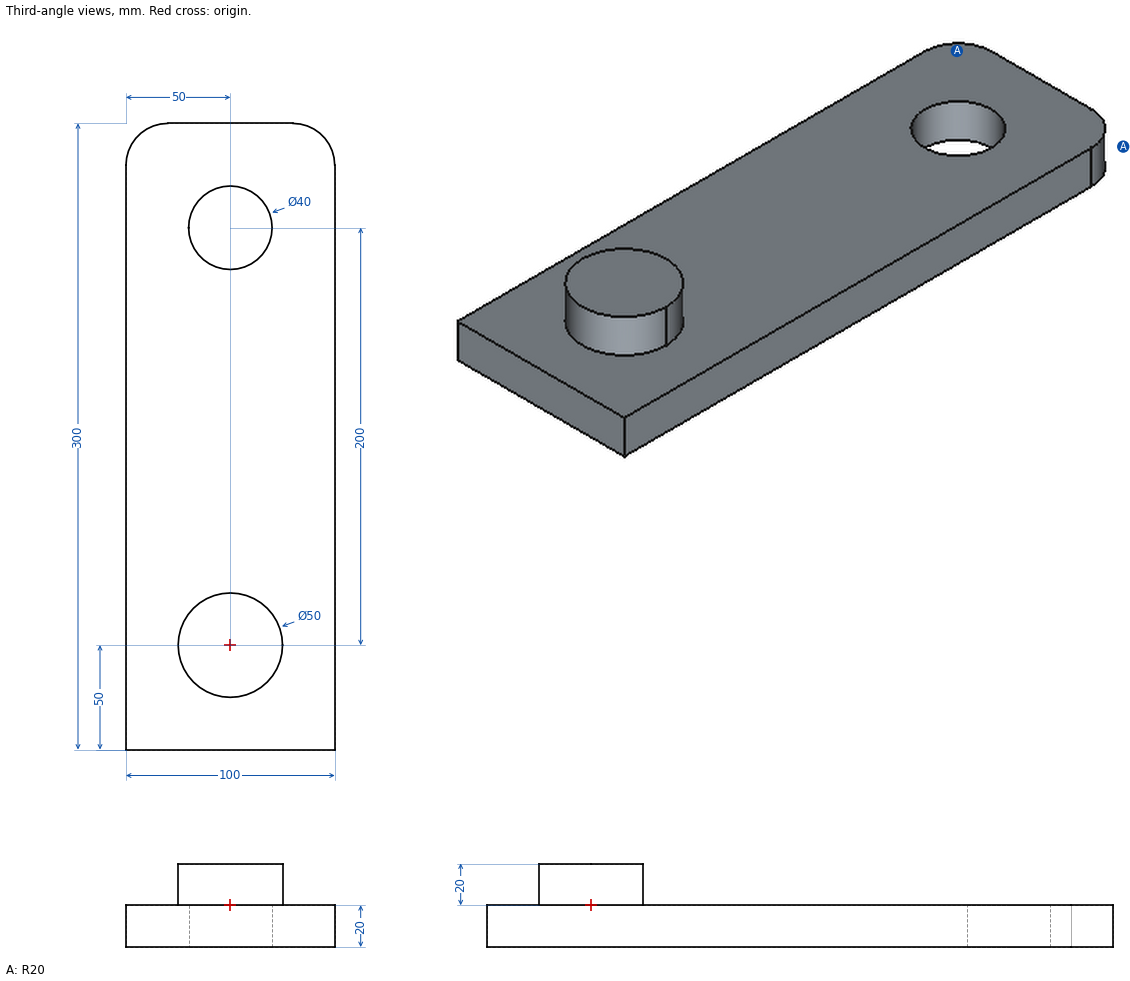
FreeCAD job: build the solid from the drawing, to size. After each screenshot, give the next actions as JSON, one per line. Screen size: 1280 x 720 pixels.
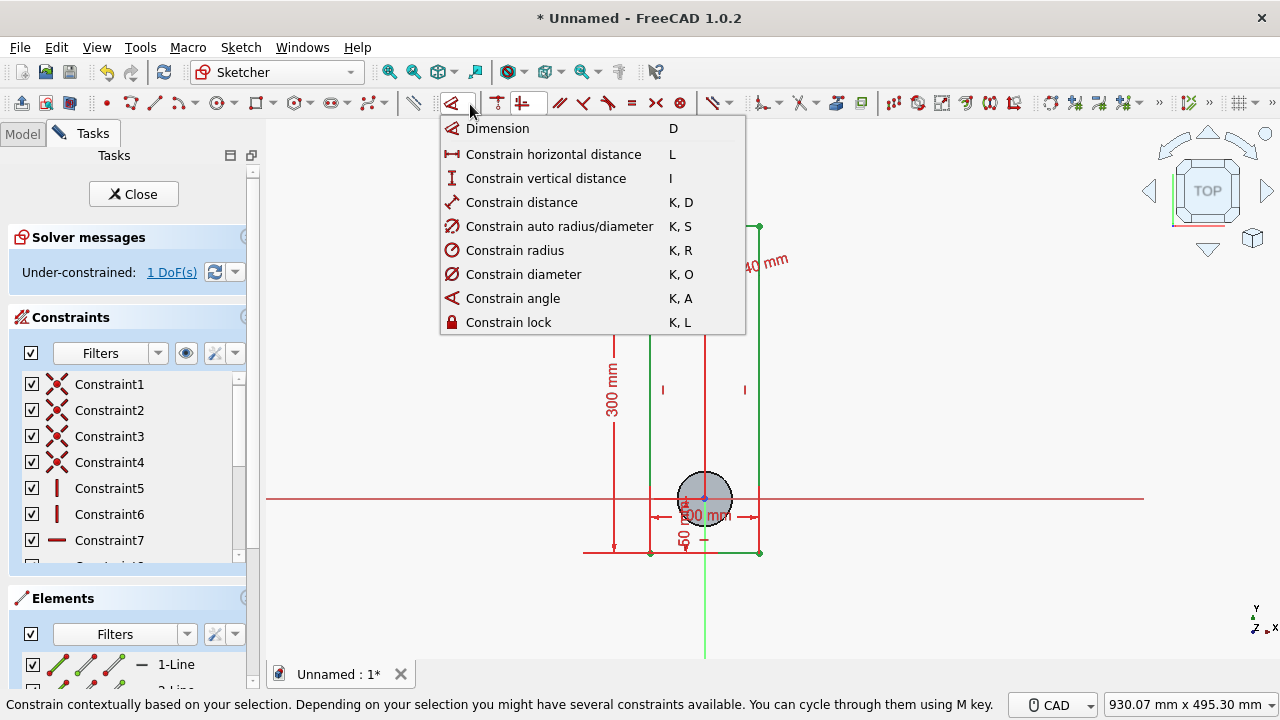
{"action": "left_click", "coordinate": [593, 178]}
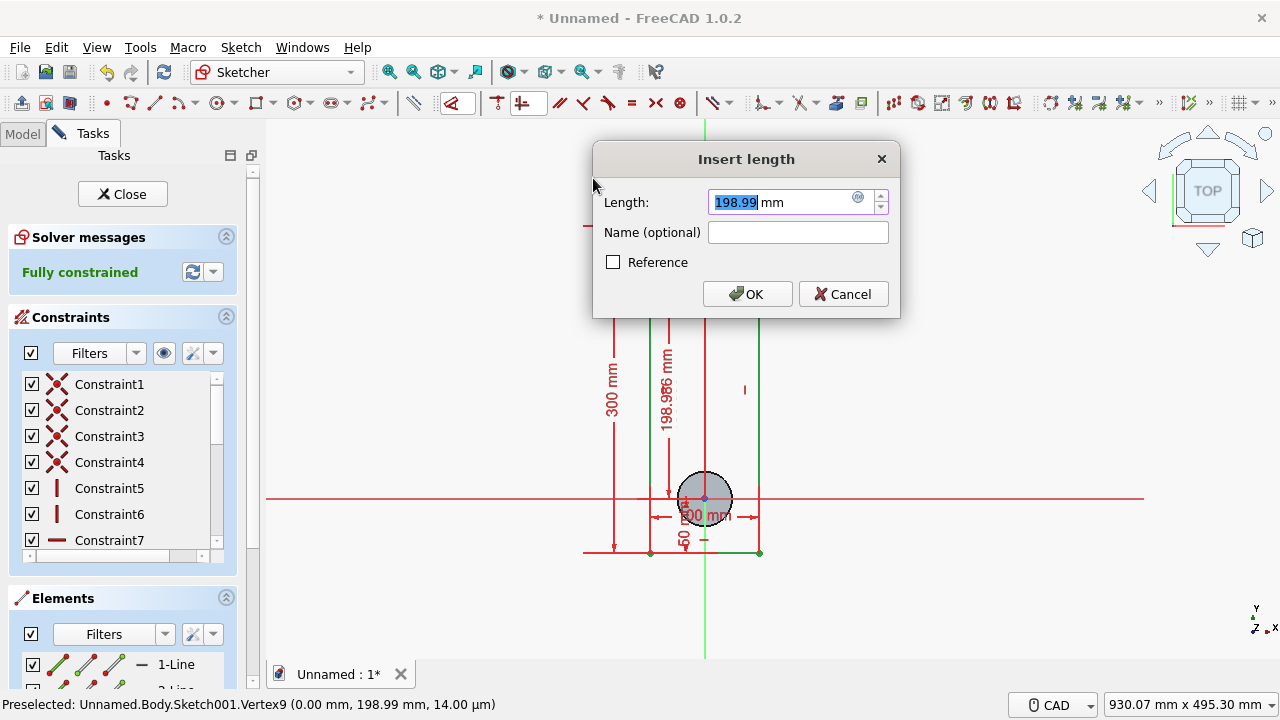
{"action": "type", "text": "200"}
{"action": "key", "text": "Return"}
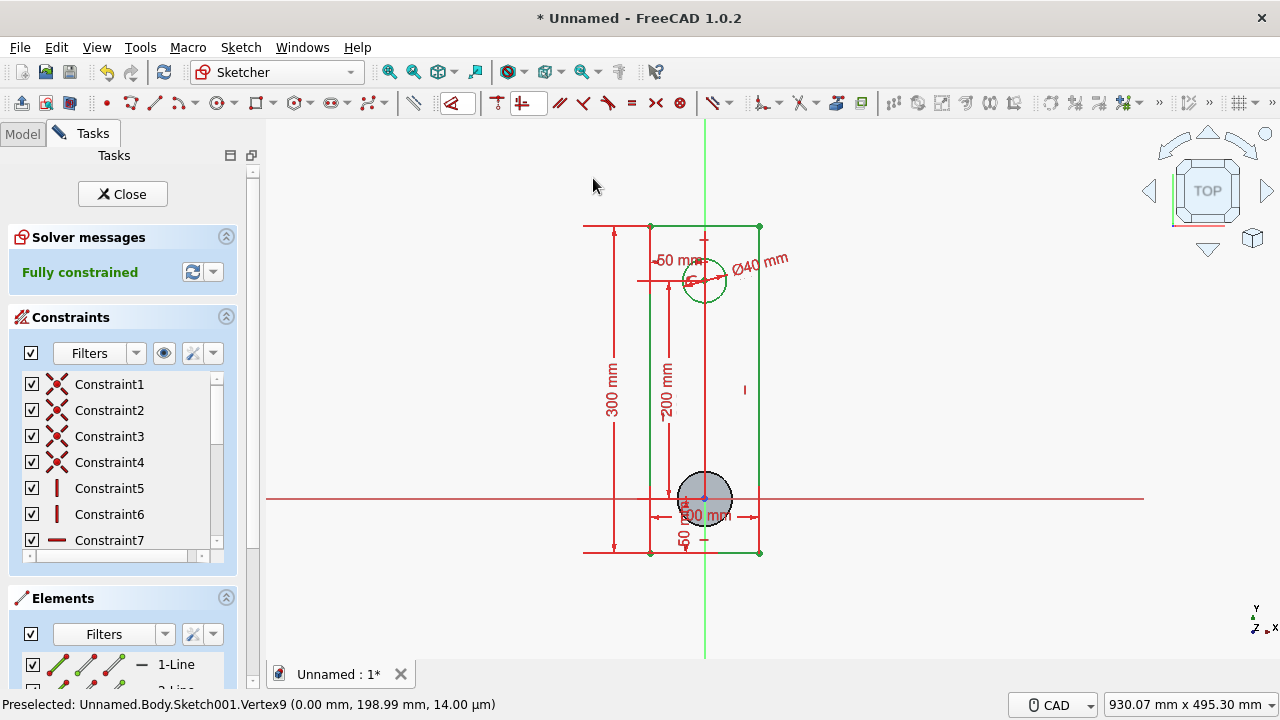
{"action": "left_click", "coordinate": [123, 194]}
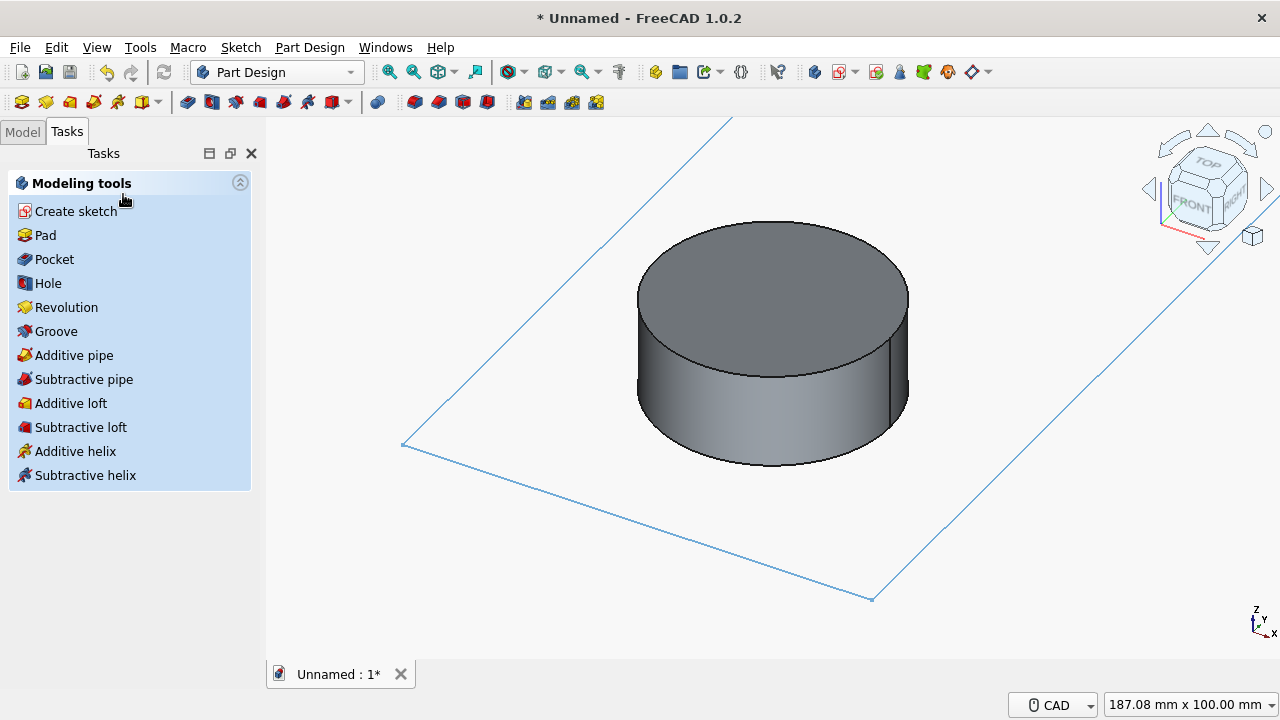
{"action": "left_click", "coordinate": [22, 102]}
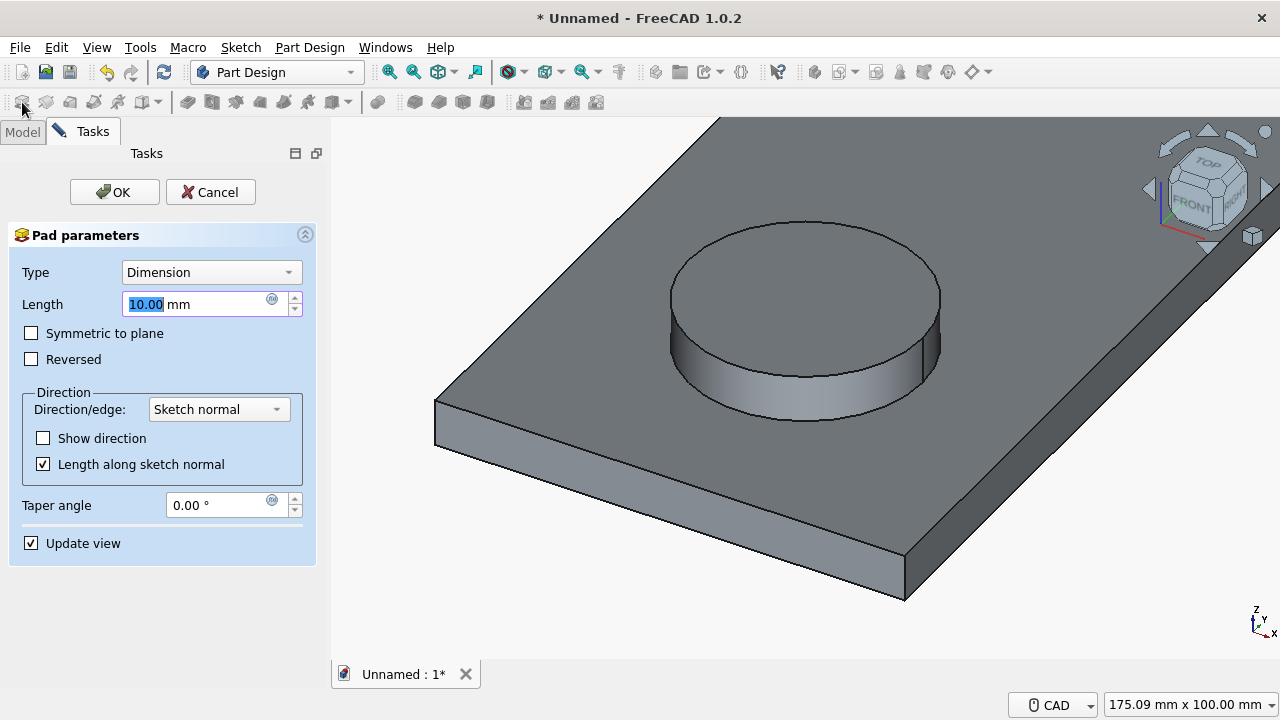
{"action": "type", "text": "20"}
{"action": "key", "text": "Tab"}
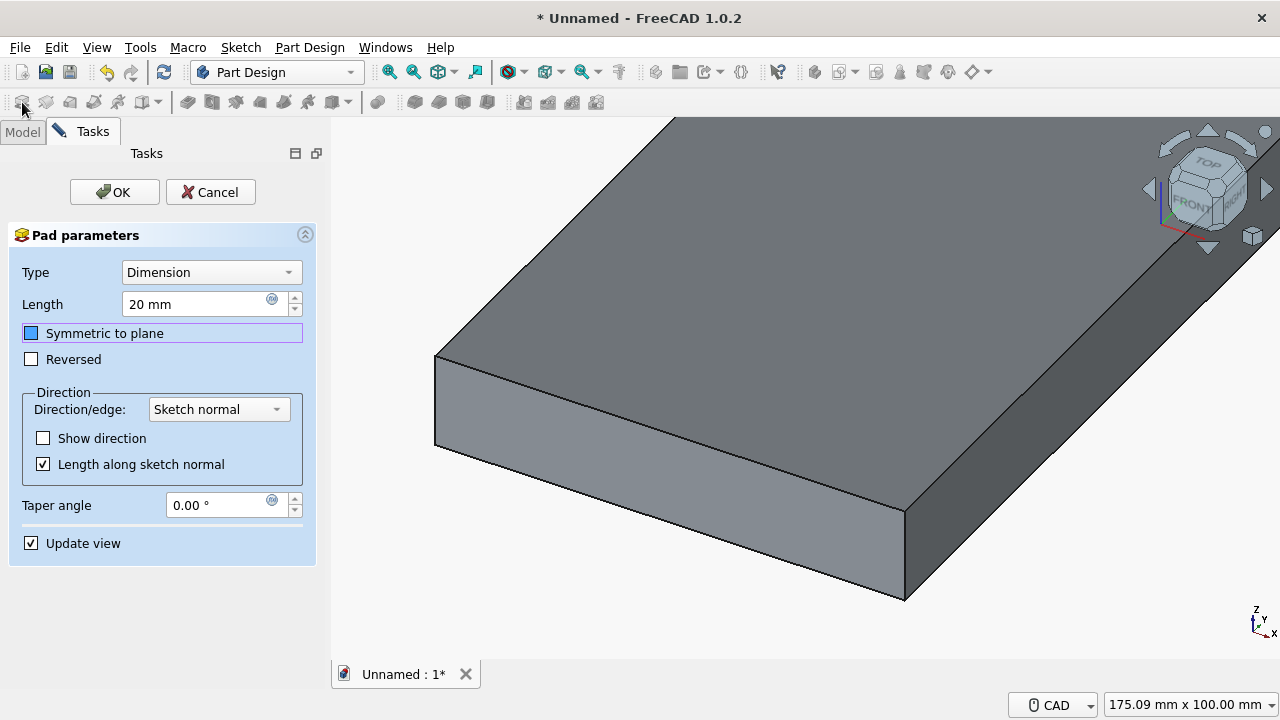
{"action": "left_click", "coordinate": [30, 359]}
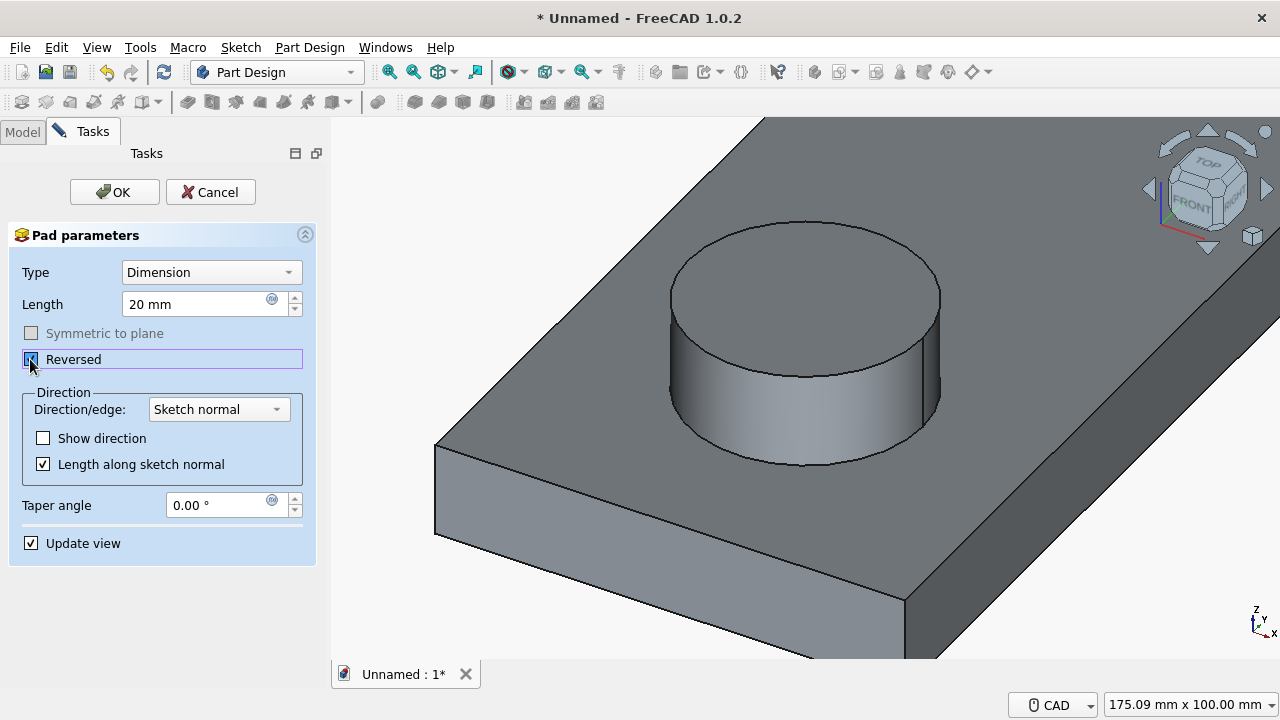
{"action": "left_click", "coordinate": [115, 192]}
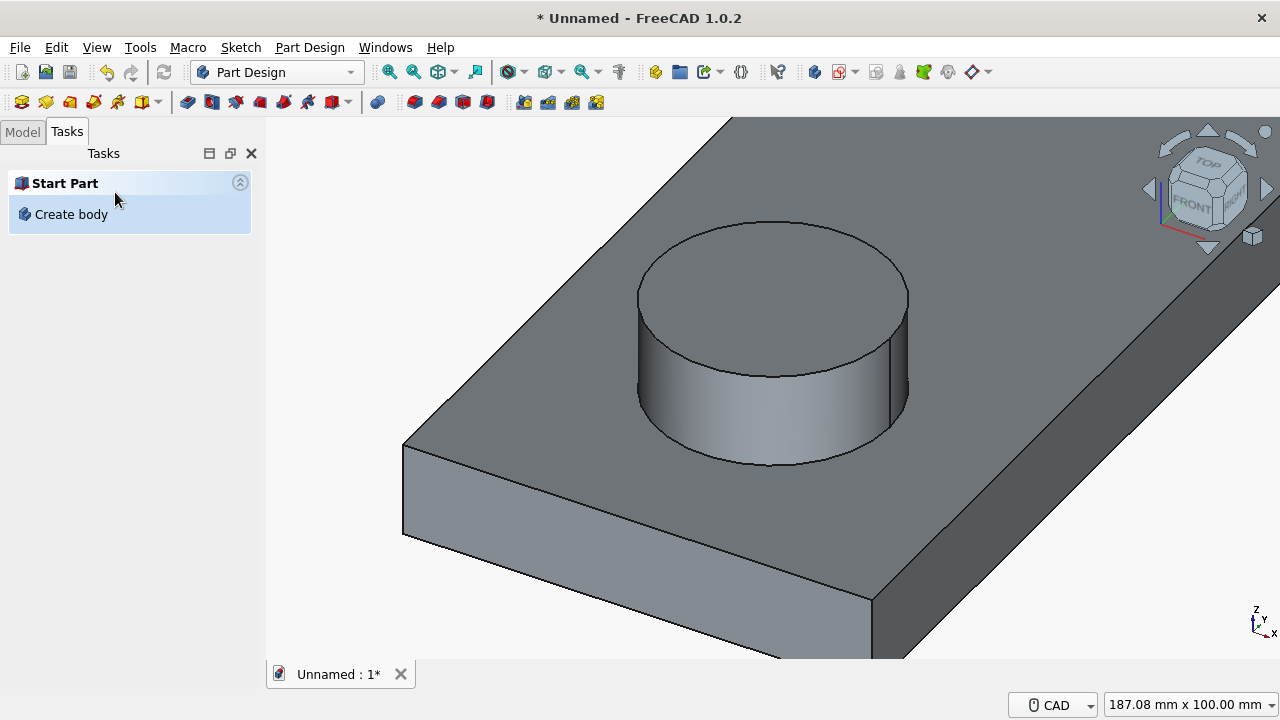
{"action": "left_click", "coordinate": [390, 72]}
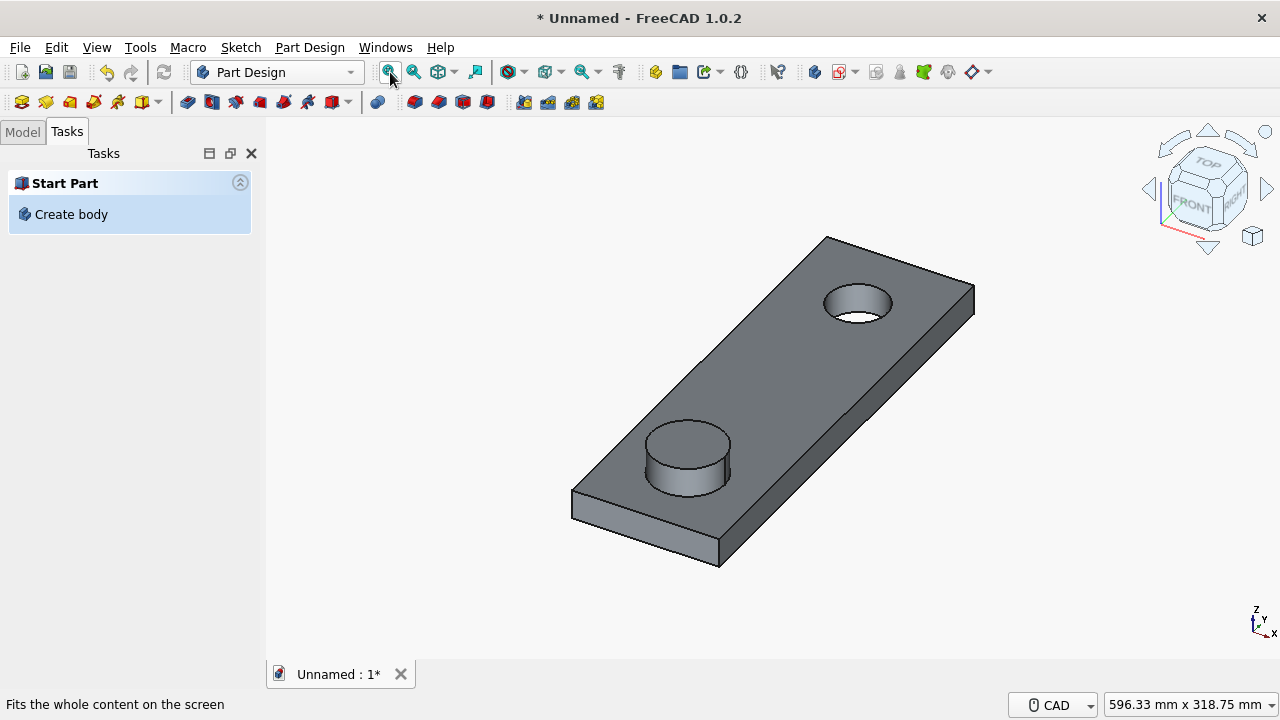
{"action": "key", "text": "0"}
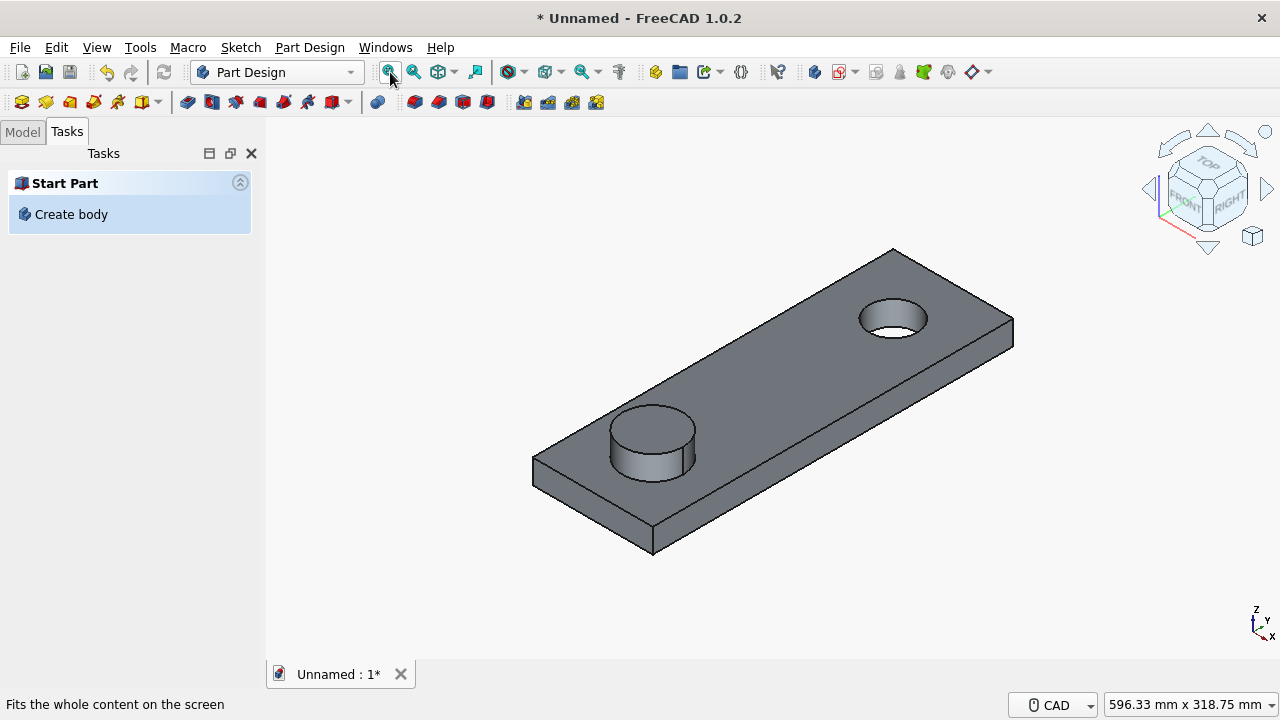
{"action": "key", "text": "2"}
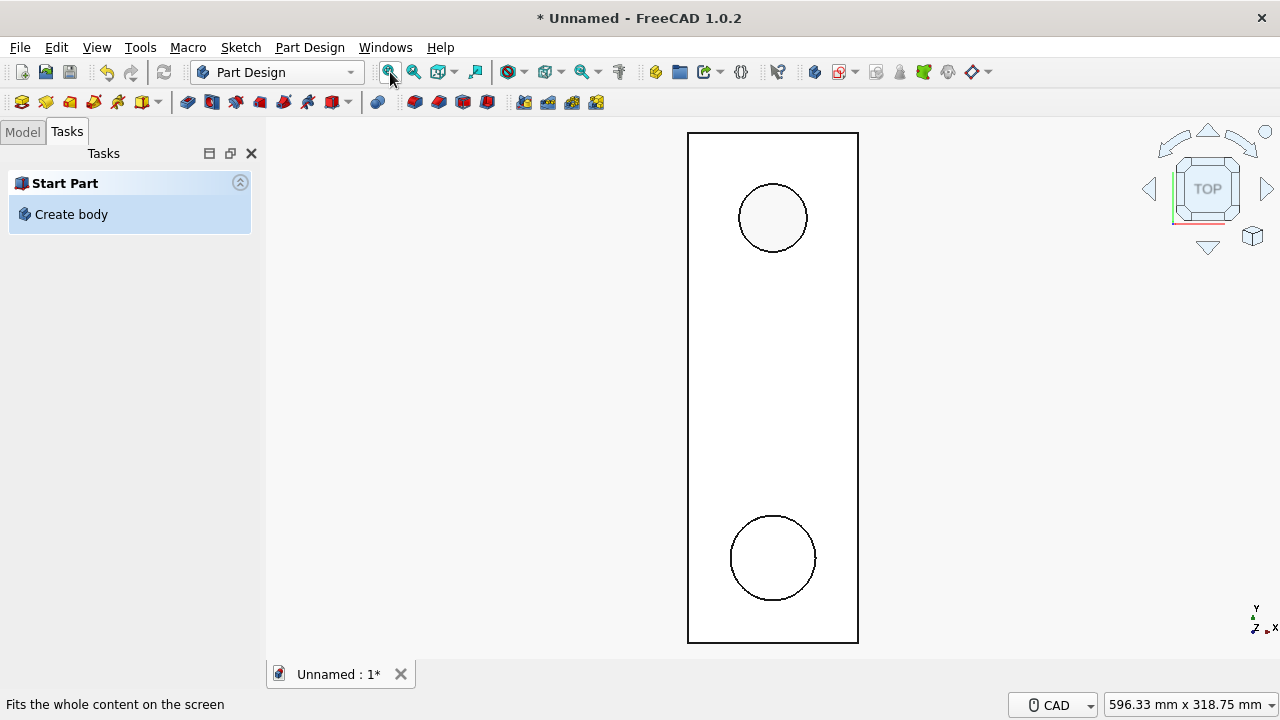
{"action": "key", "text": "1"}